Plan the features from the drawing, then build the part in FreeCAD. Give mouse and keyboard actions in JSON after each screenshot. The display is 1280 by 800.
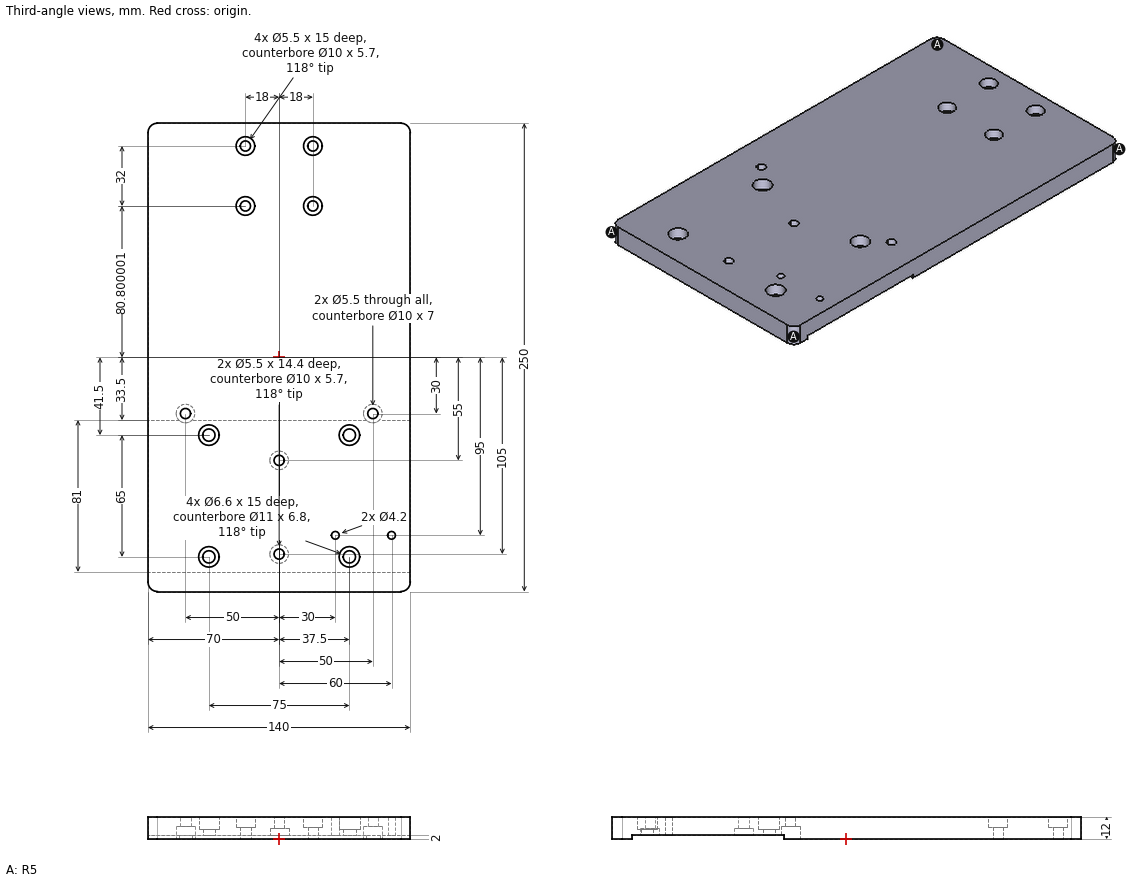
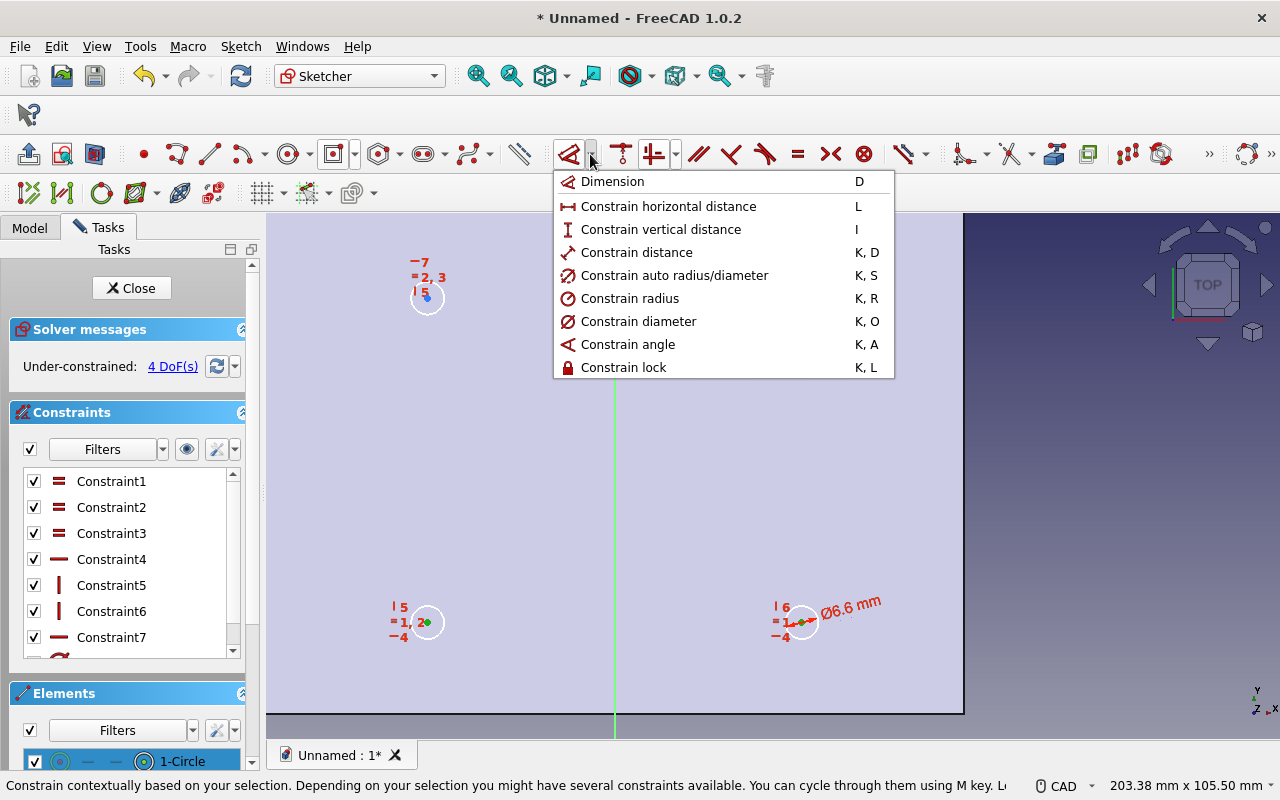
{"action": "left_click", "coordinate": [724, 206]}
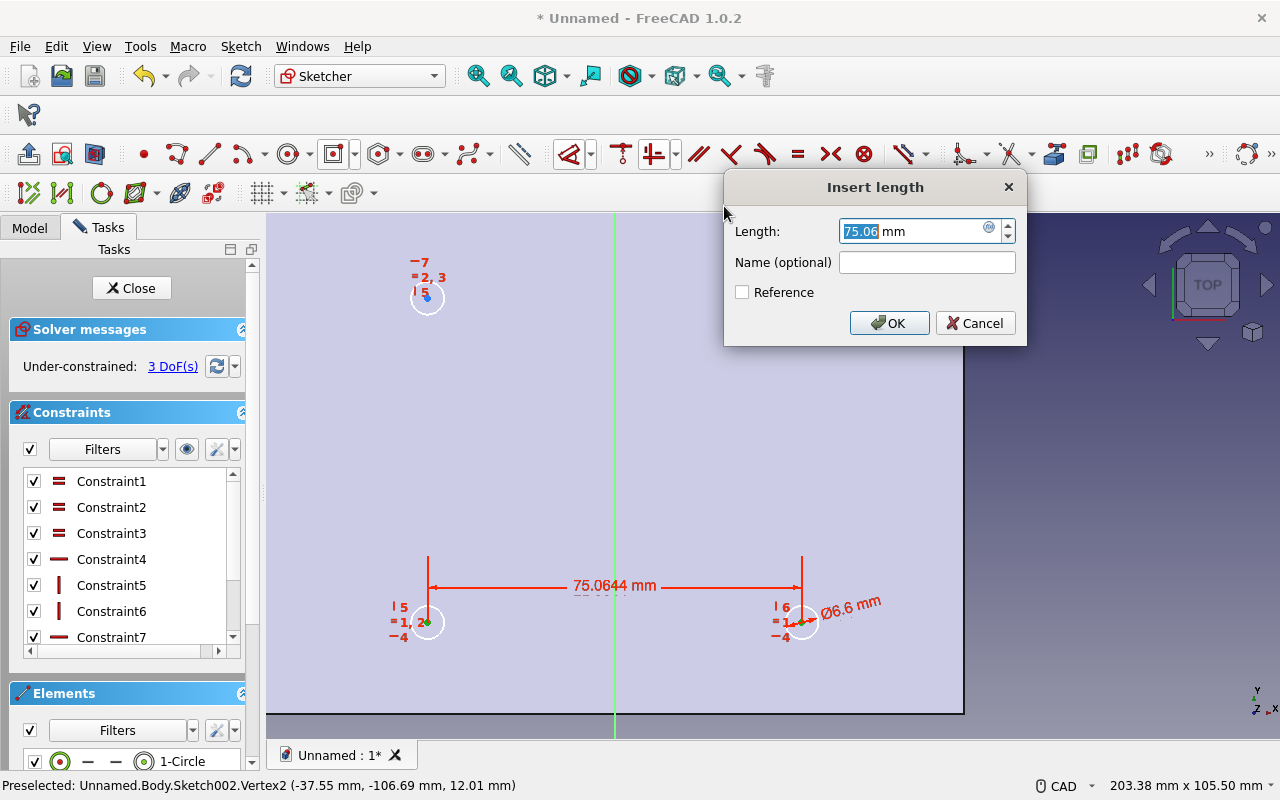
{"action": "type", "text": "75"}
{"action": "key", "text": "Return"}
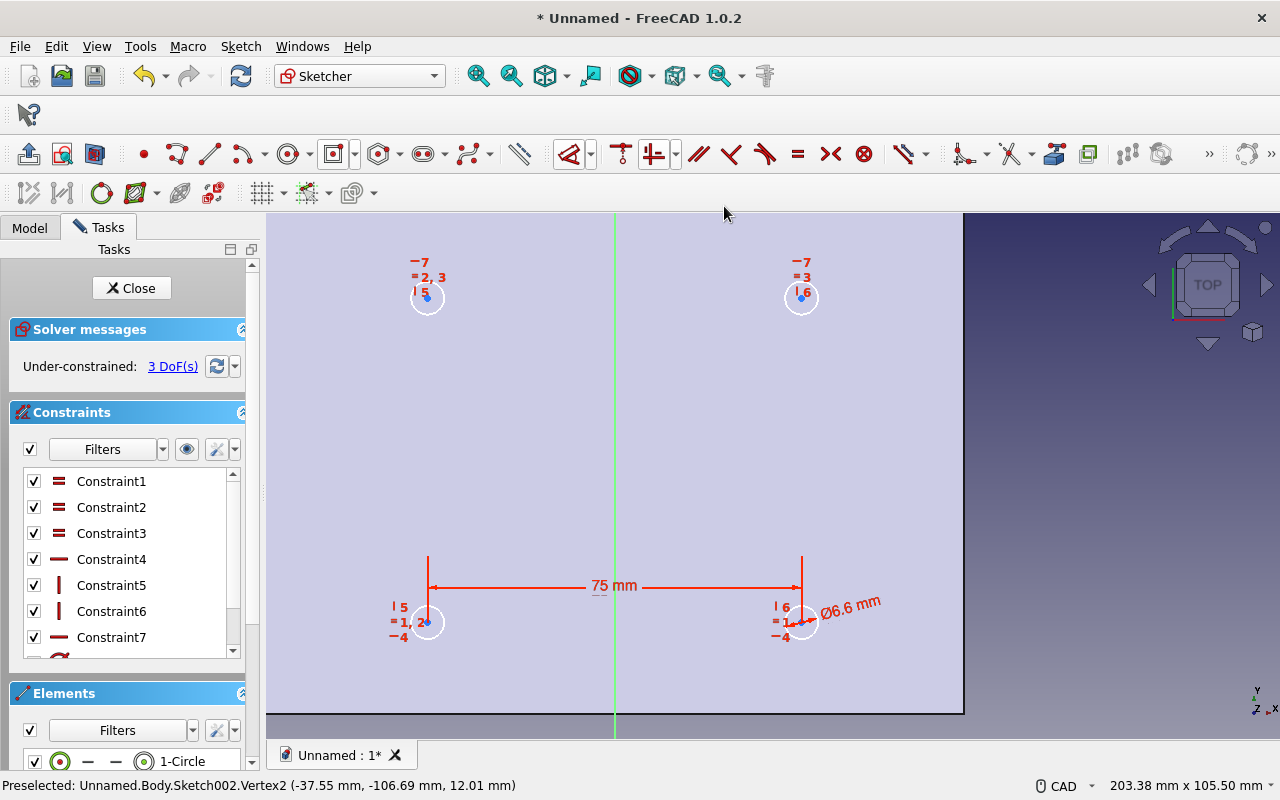
{"action": "left_click", "coordinate": [428, 623]}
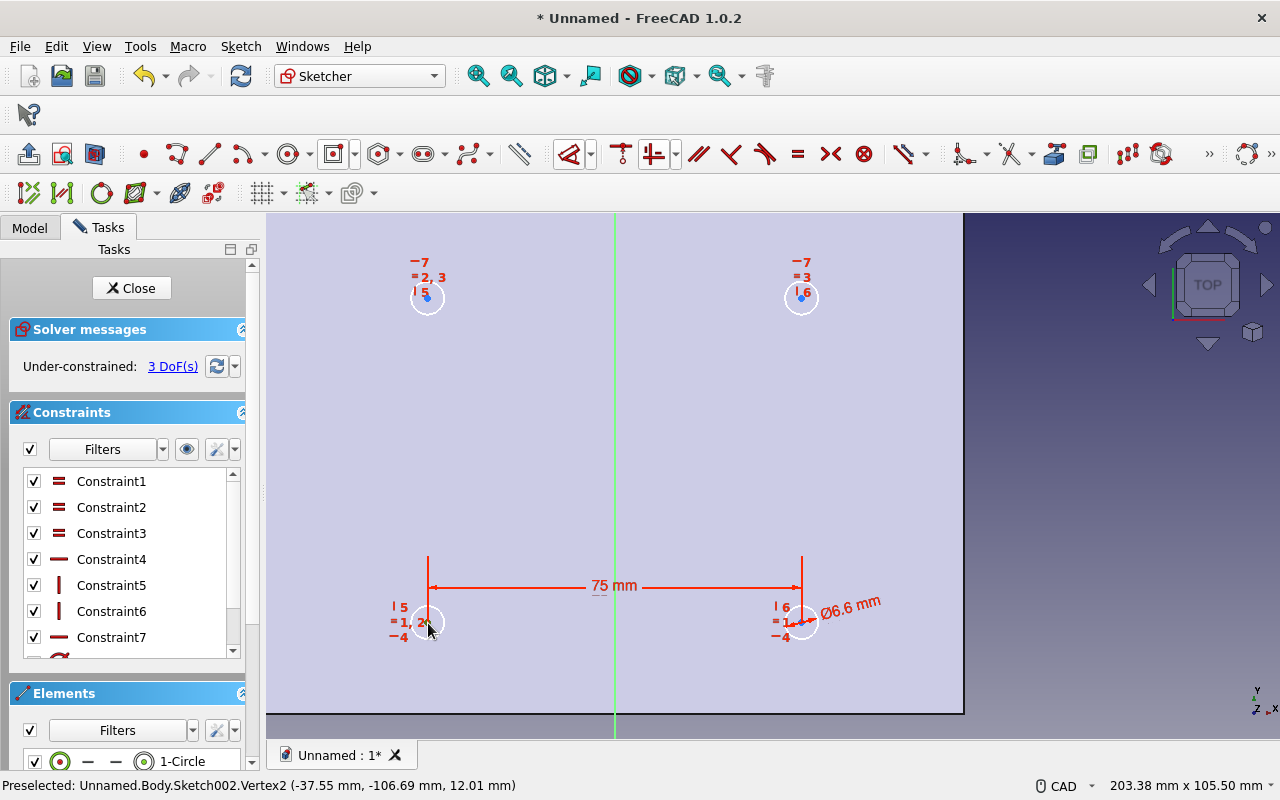
{"action": "left_click", "coordinate": [428, 298]}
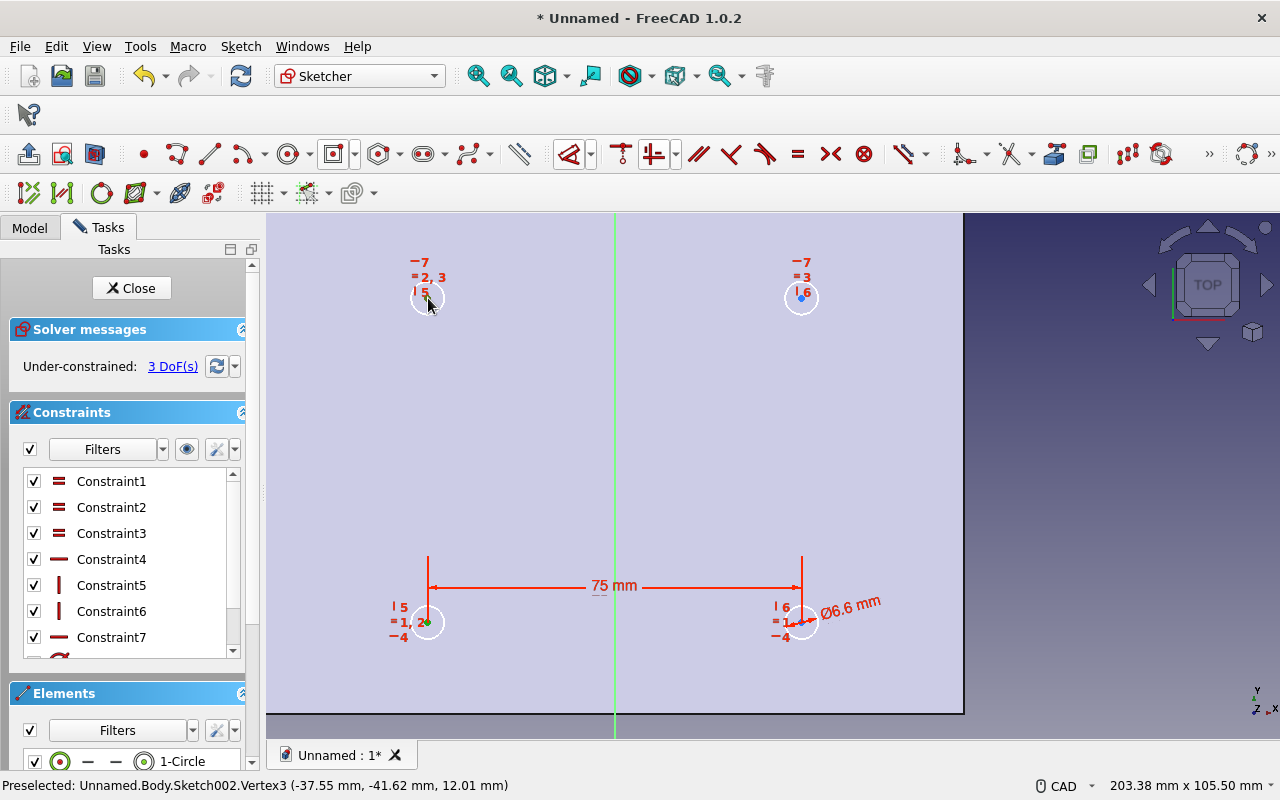
{"action": "left_click", "coordinate": [590, 154]}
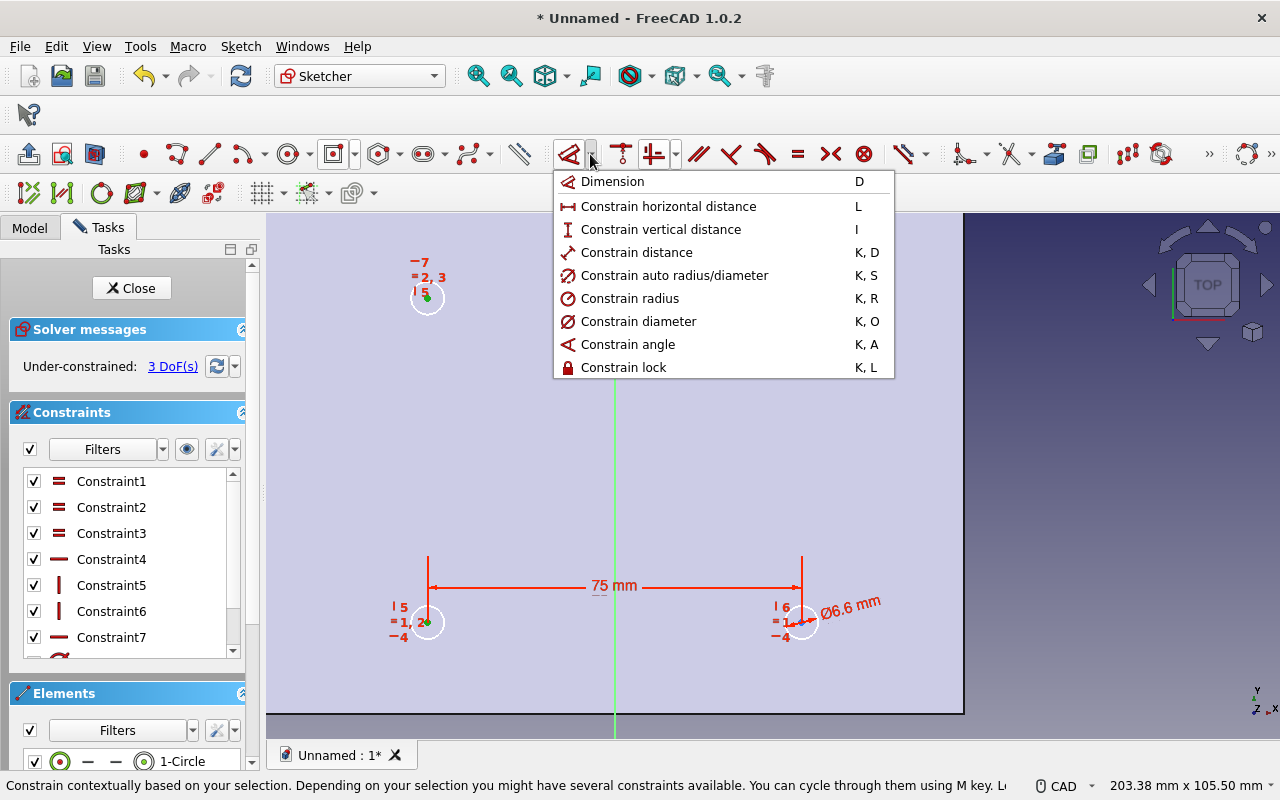
{"action": "left_click", "coordinate": [724, 230]}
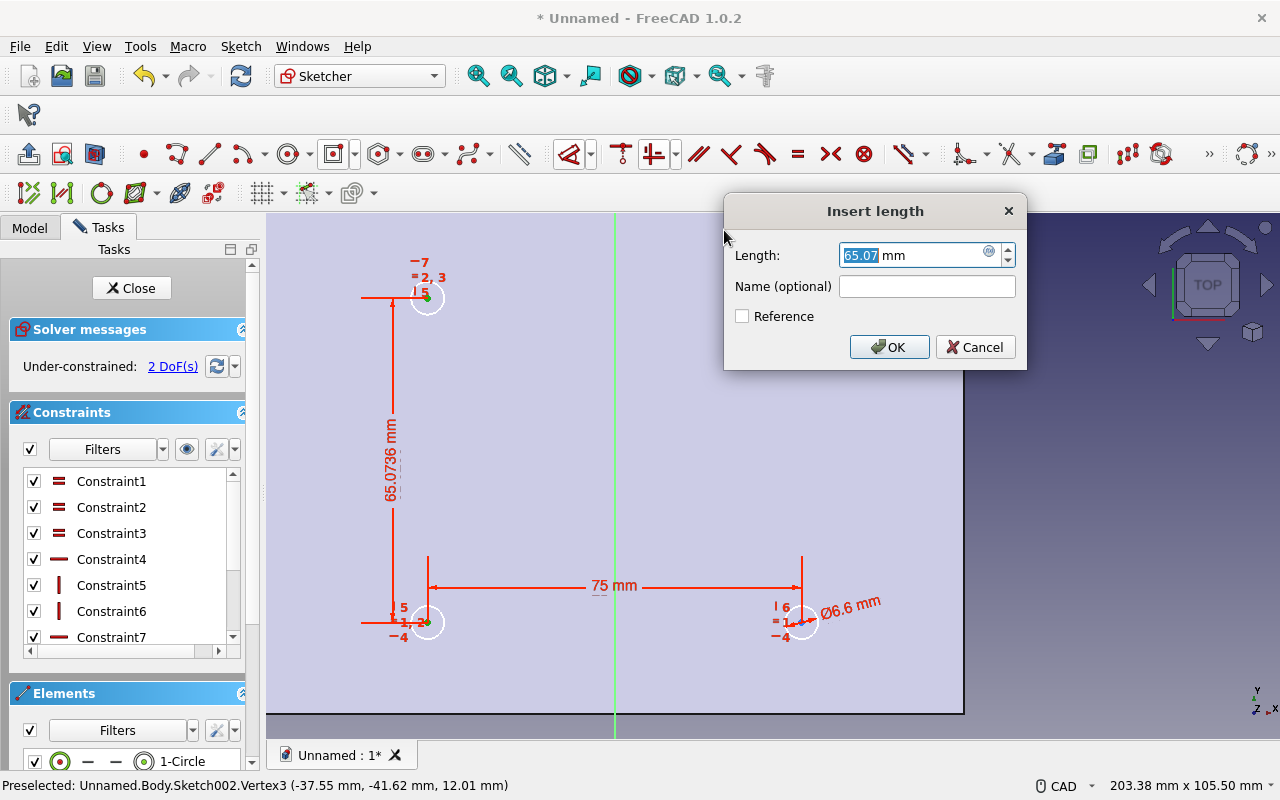
{"action": "type", "text": "65"}
{"action": "key", "text": "Return"}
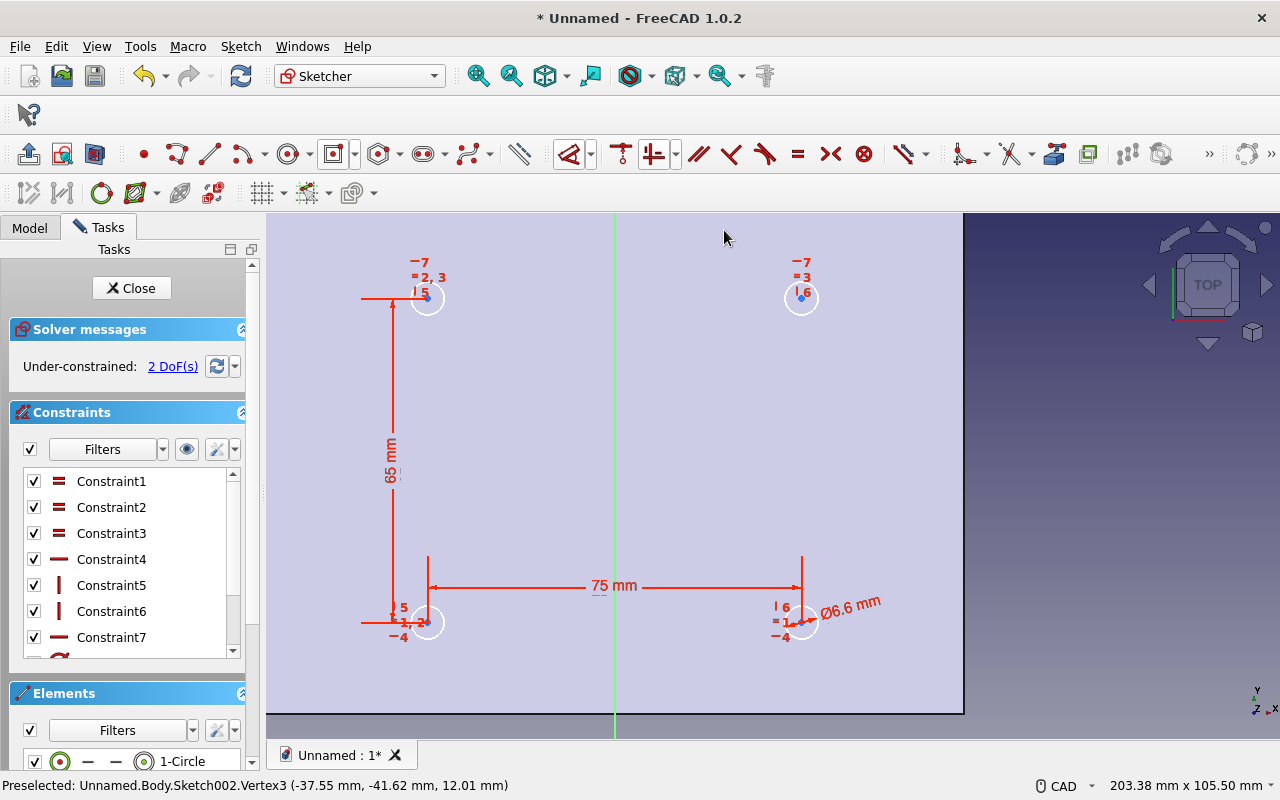
{"action": "left_click", "coordinate": [802, 623]}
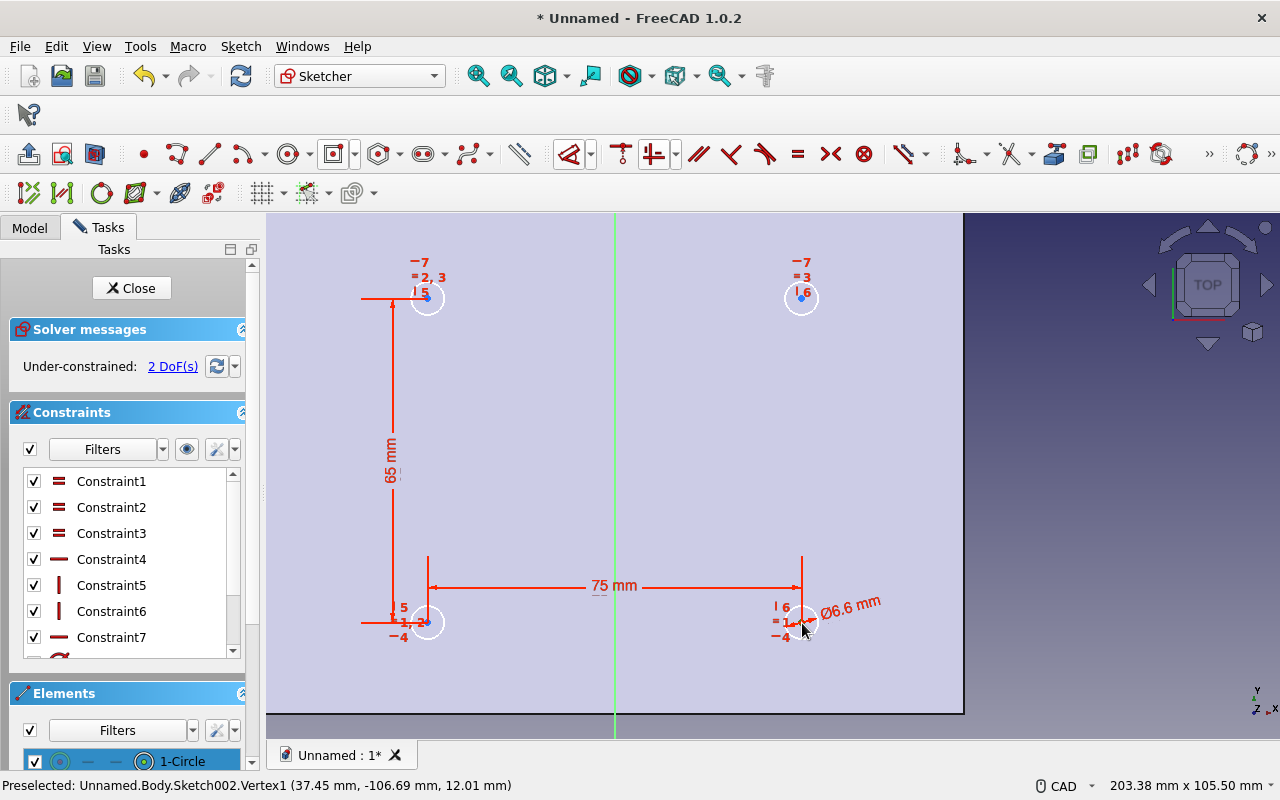
{"action": "key", "text": "l"}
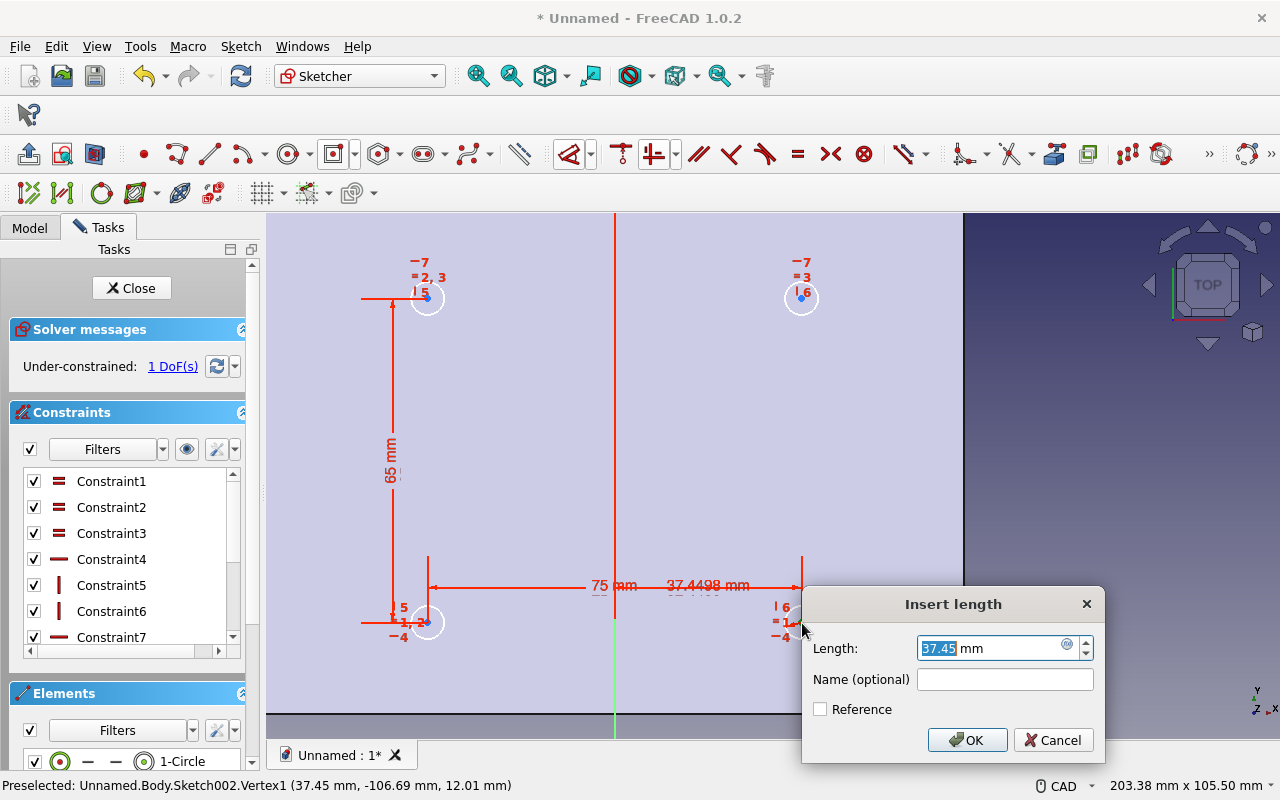
{"action": "type", "text": "37.5"}
{"action": "key", "text": "Return"}